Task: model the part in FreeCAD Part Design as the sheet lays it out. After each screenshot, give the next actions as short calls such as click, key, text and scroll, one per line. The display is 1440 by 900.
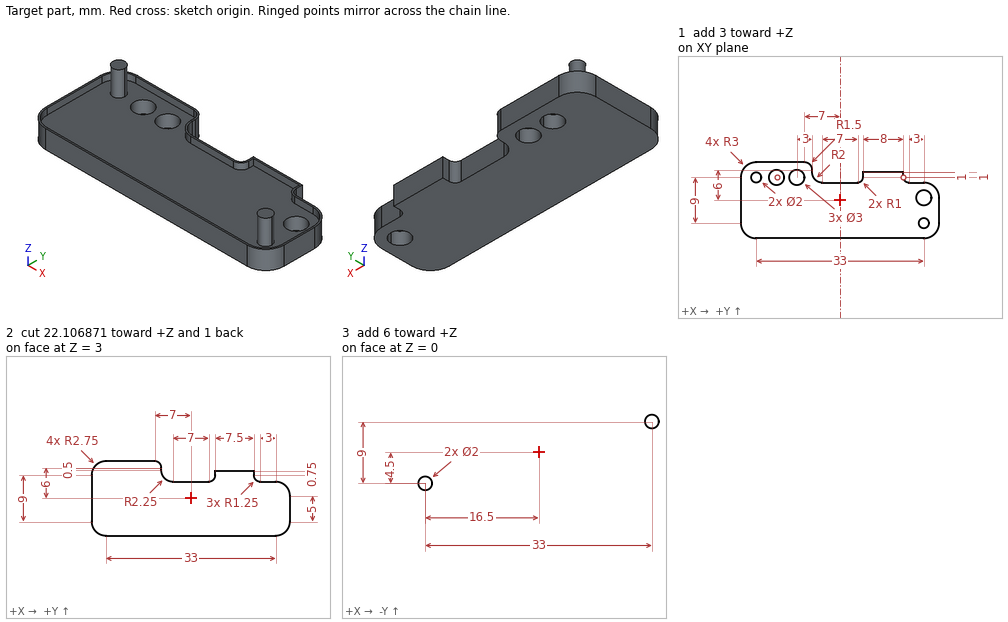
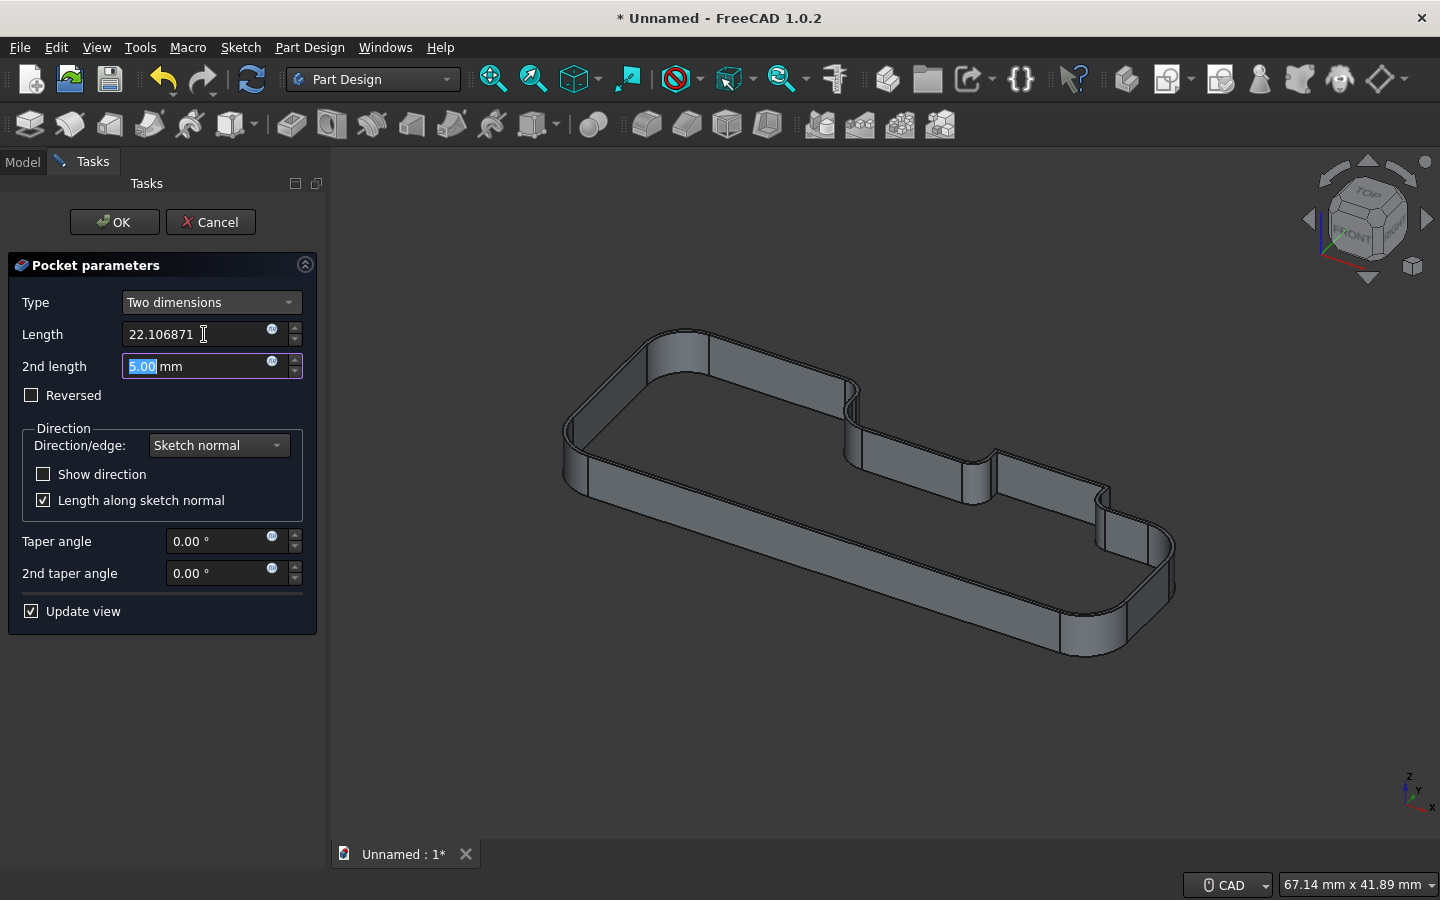
text(1)
key(Tab)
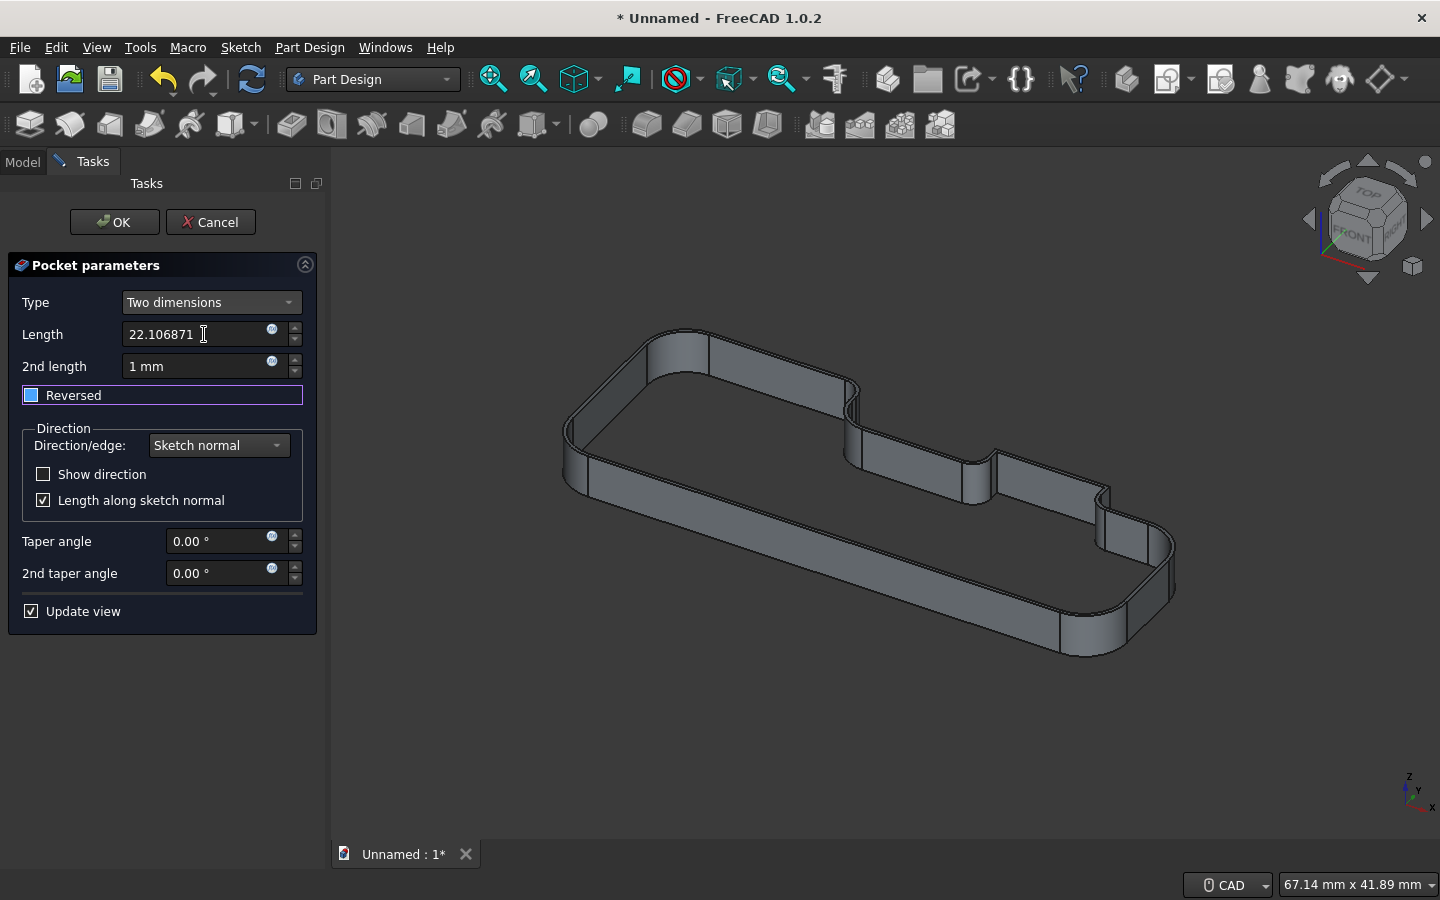
click(30, 395)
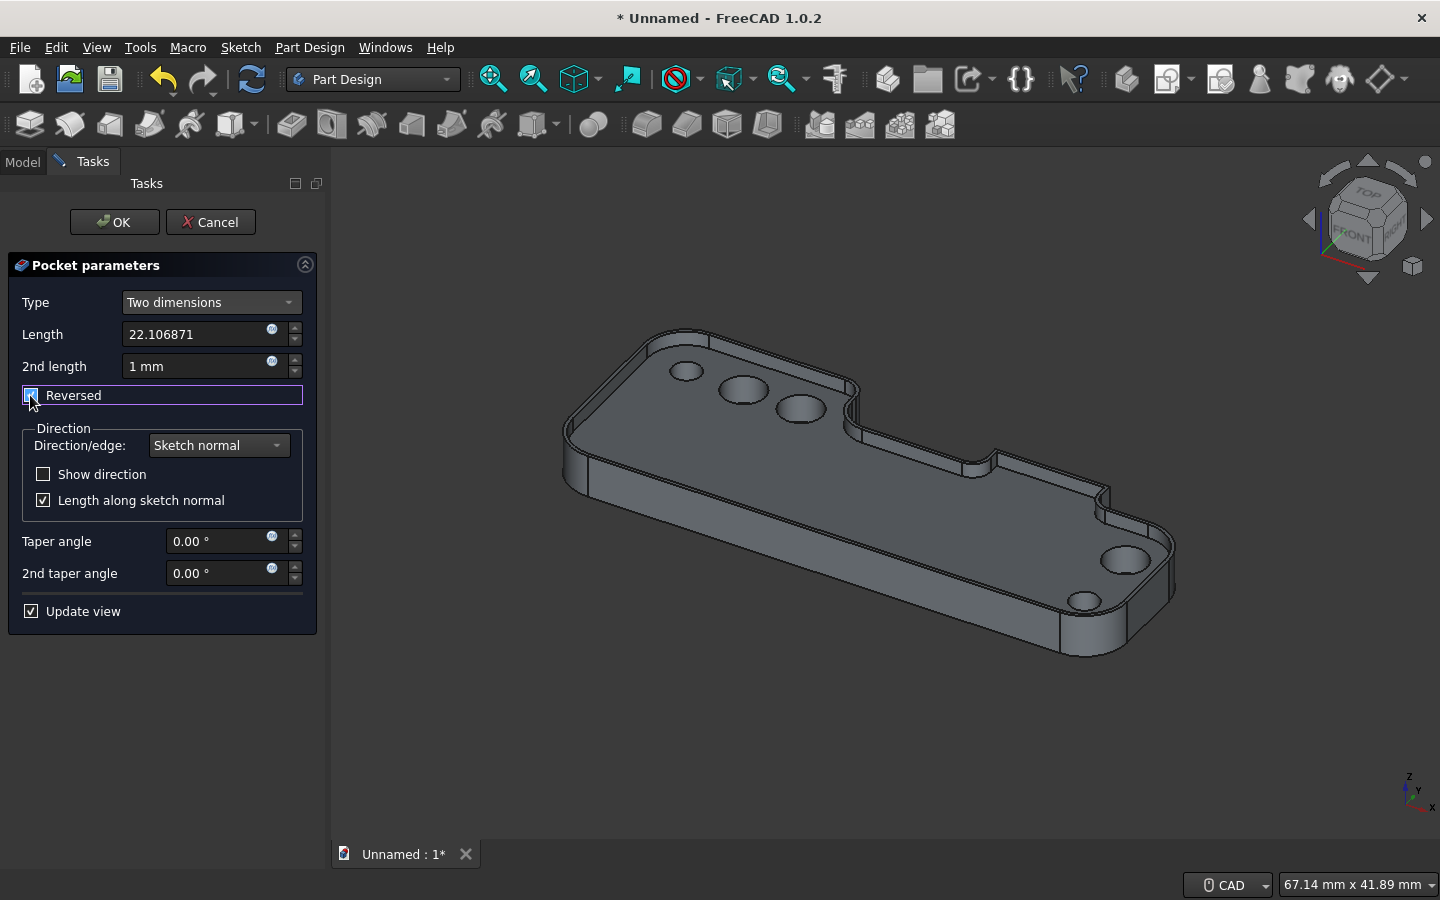
click(115, 222)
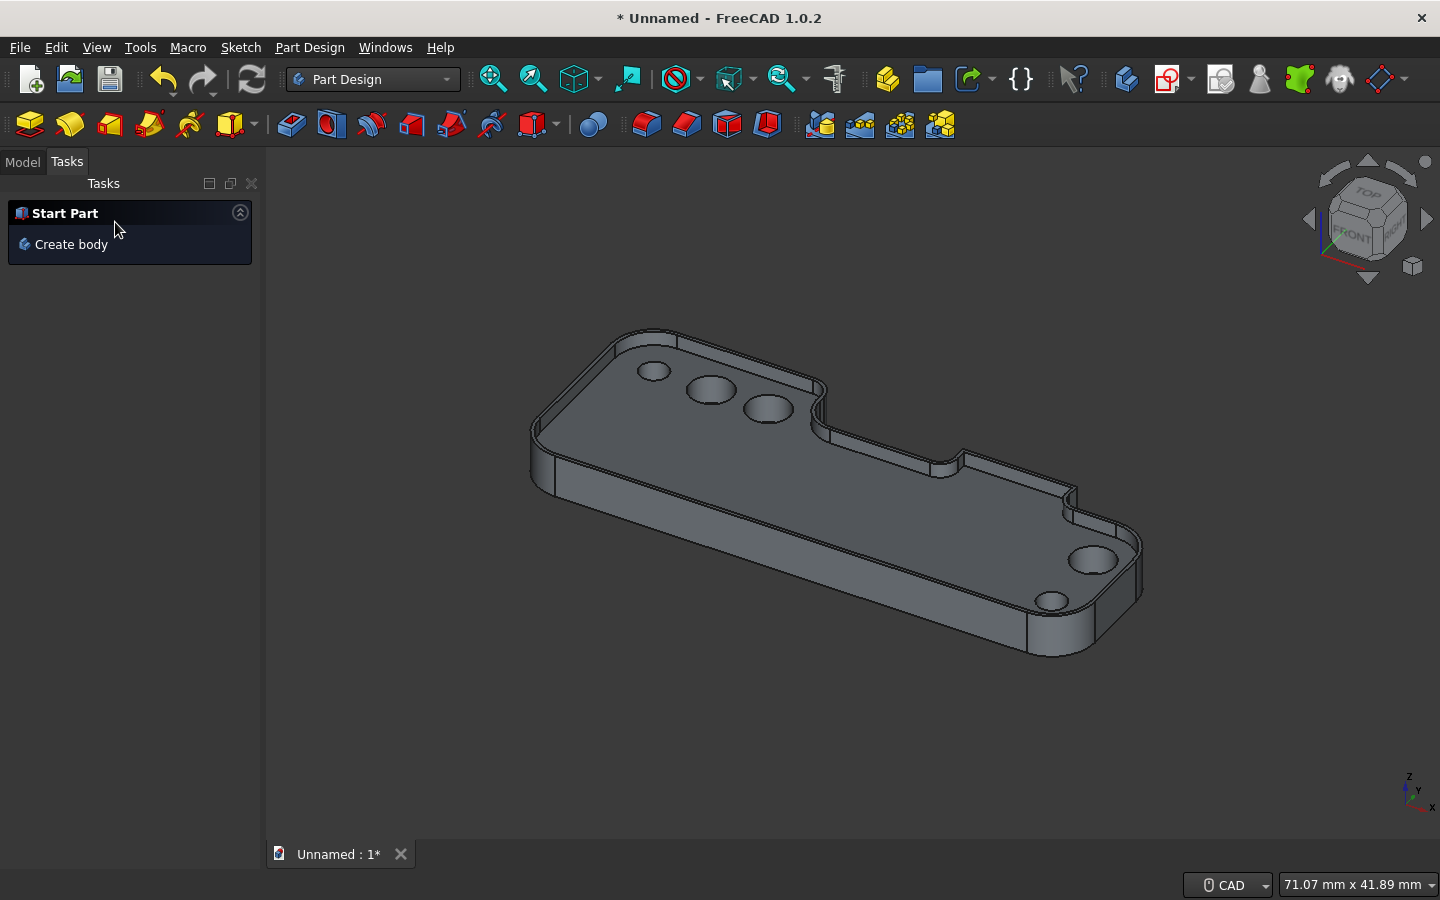
key(5)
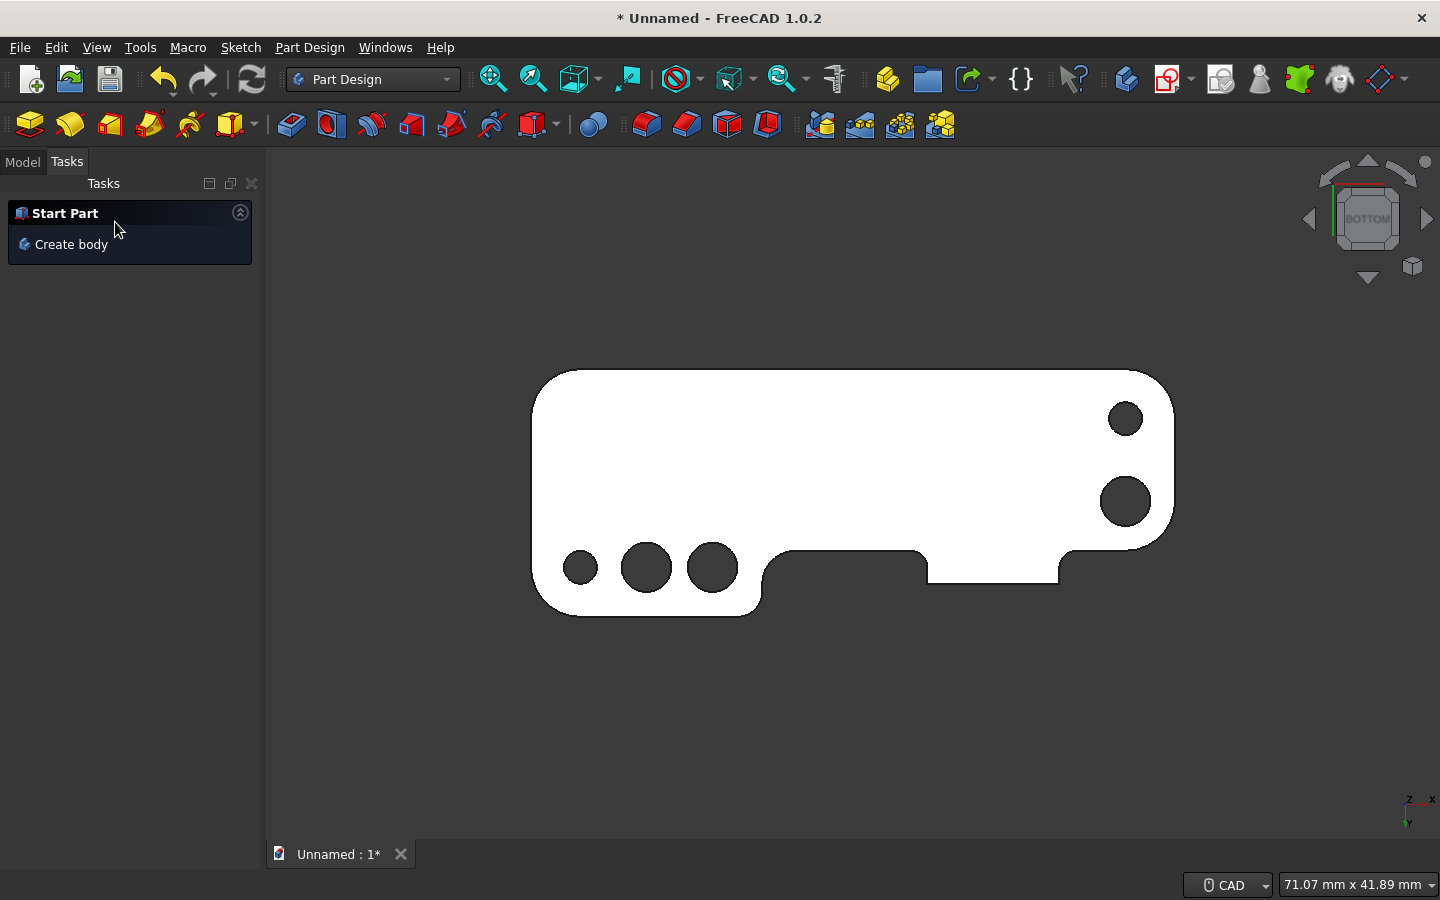
click(945, 457)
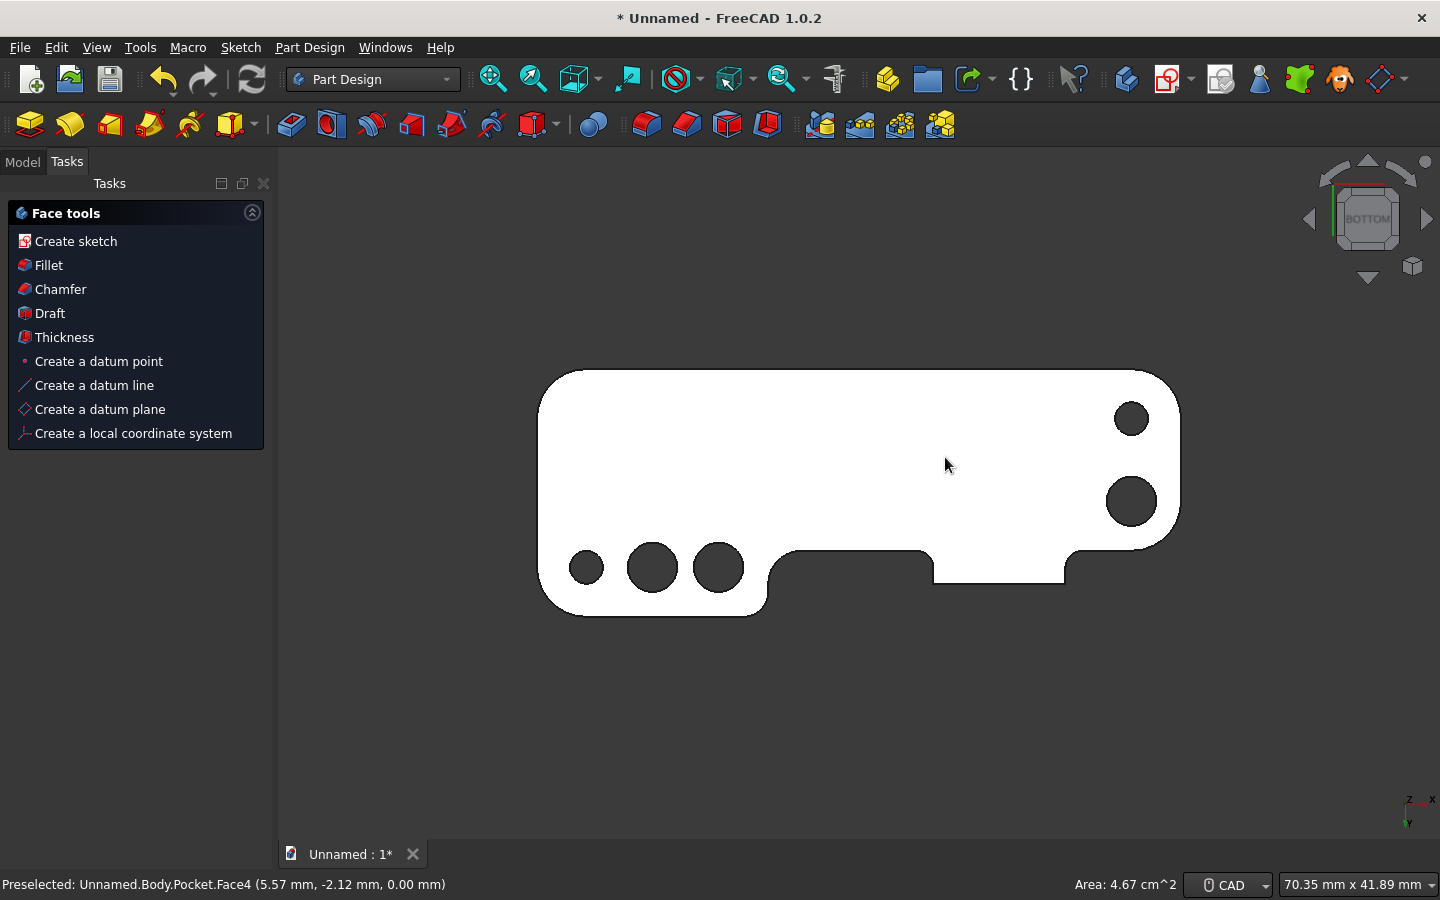
click(1168, 80)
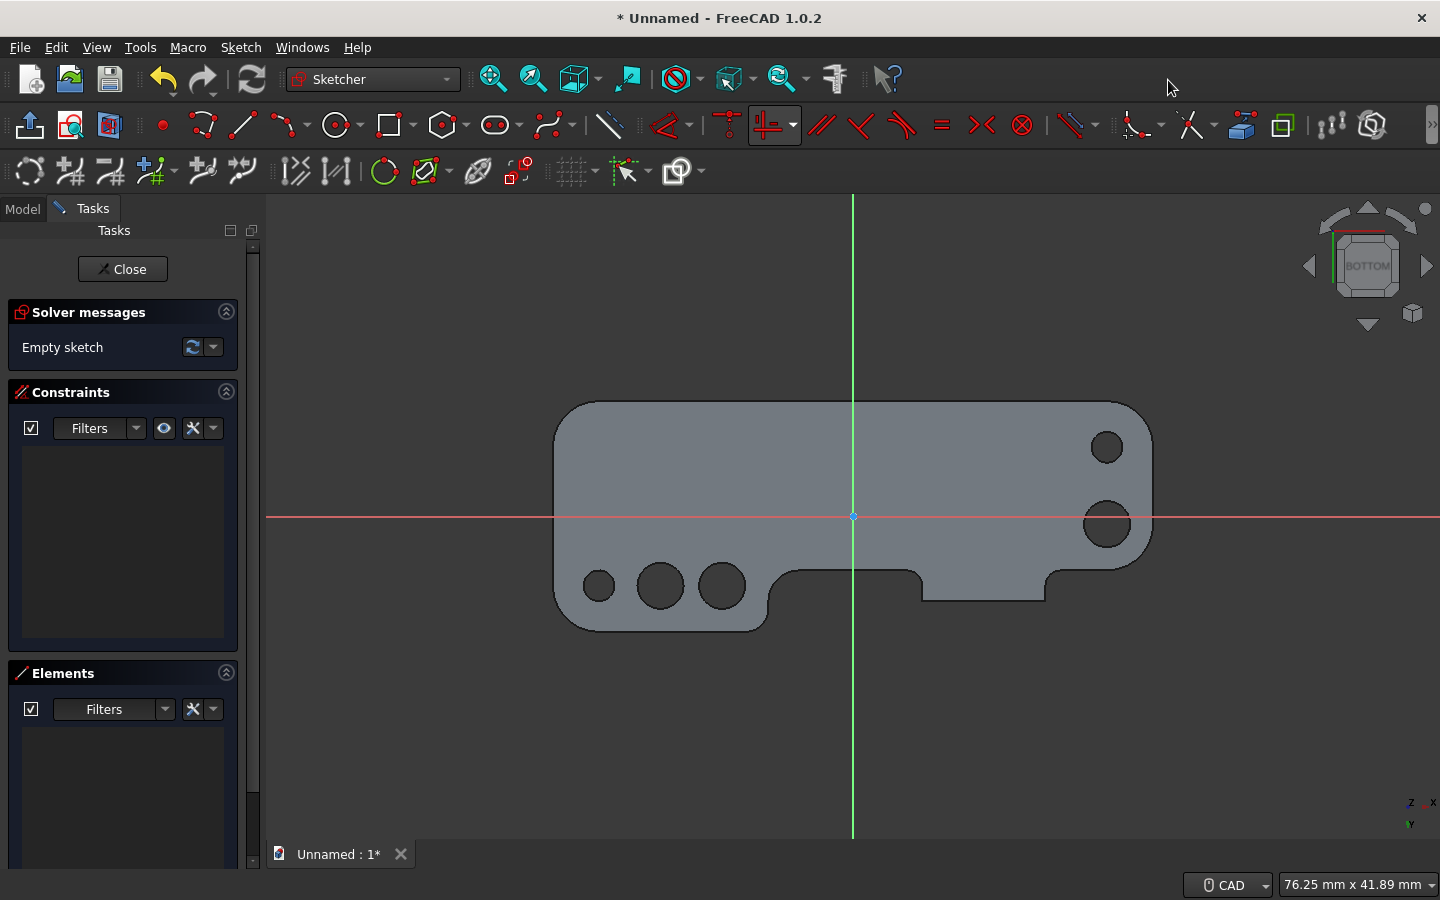
click(336, 126)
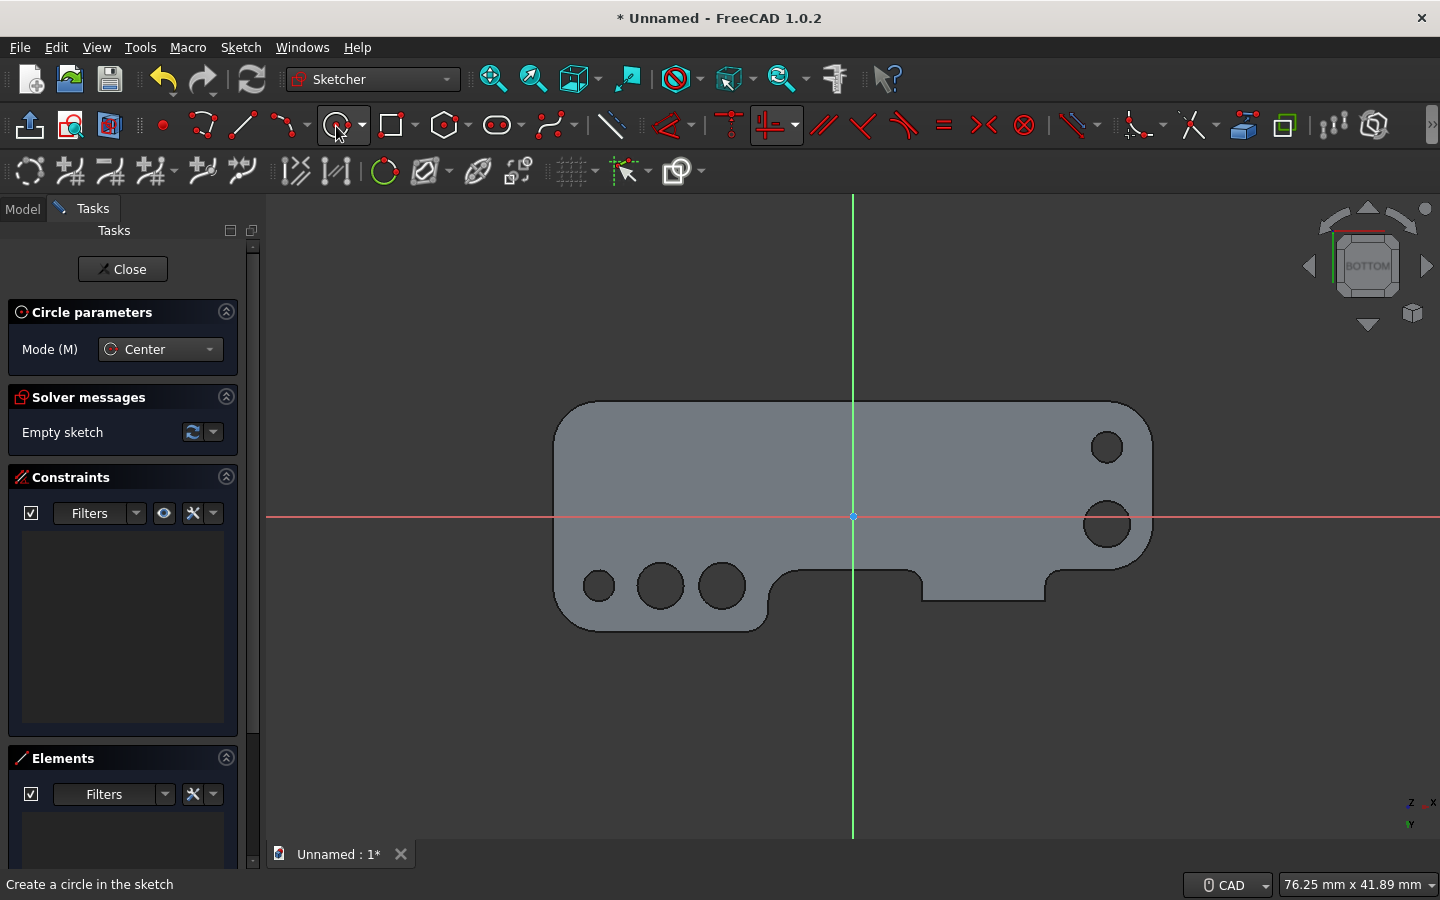
scroll(599, 586, up, 2)